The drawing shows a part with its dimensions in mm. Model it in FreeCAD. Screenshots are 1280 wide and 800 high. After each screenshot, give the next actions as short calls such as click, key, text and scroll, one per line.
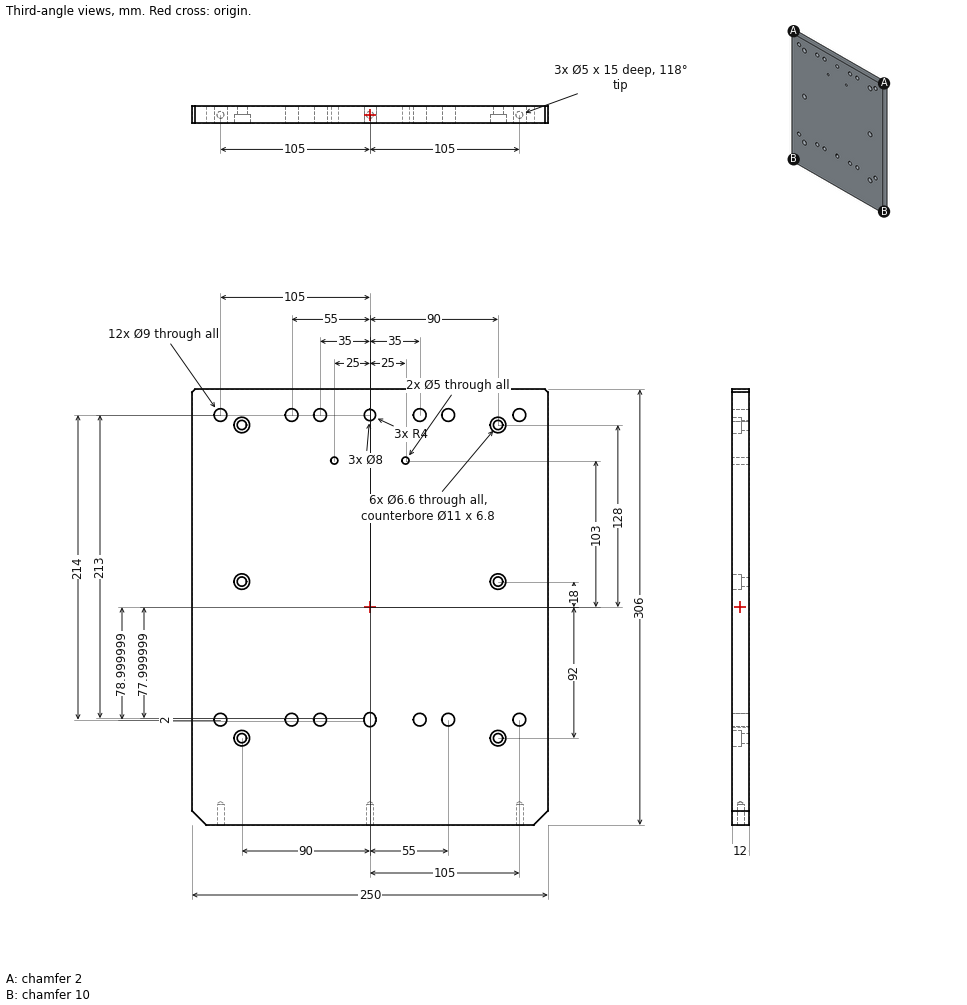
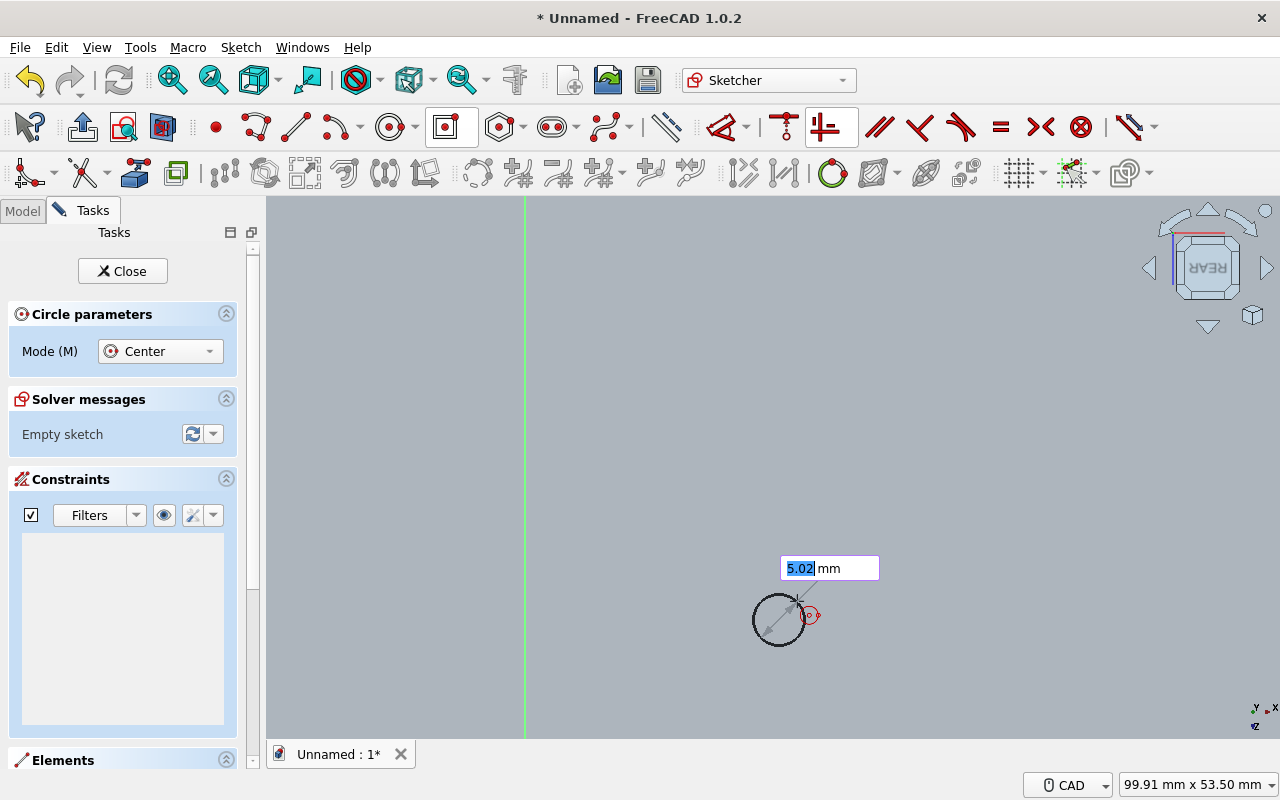
text(5)
key(Return)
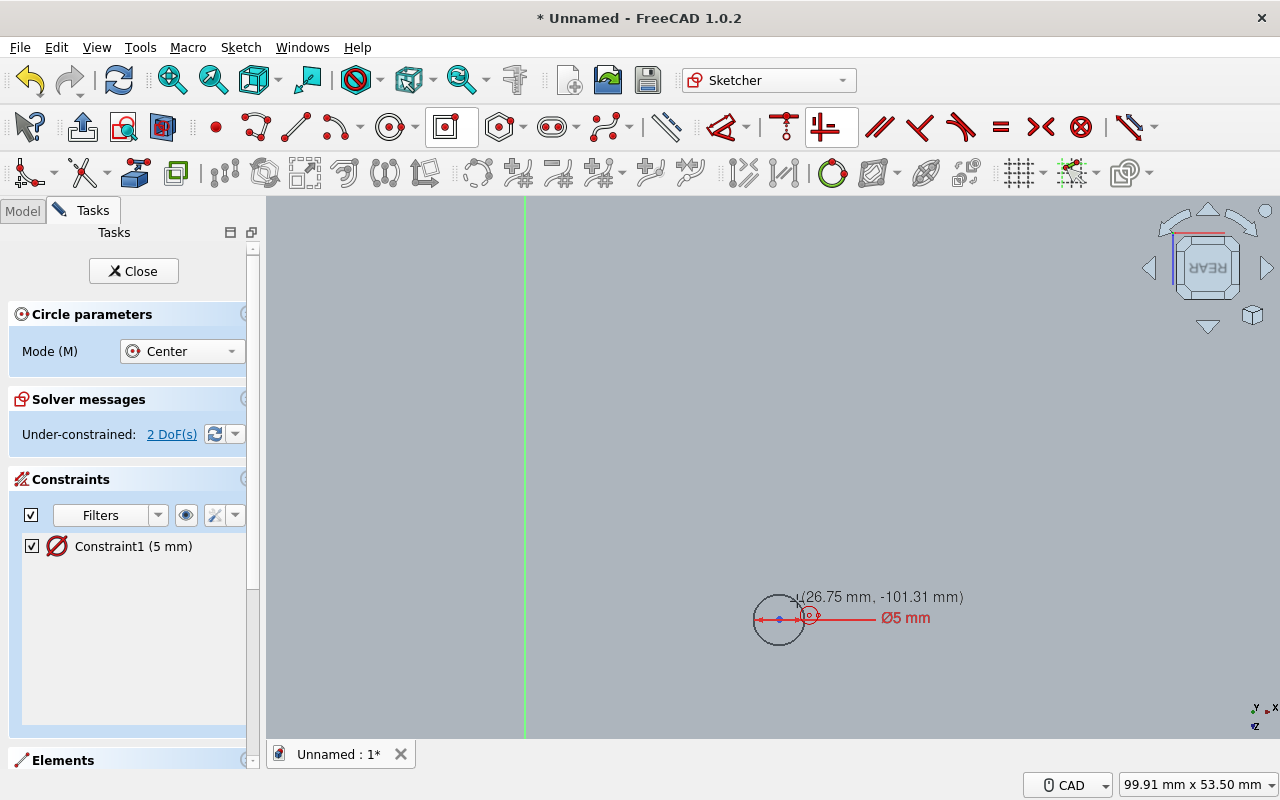
scroll(782, 622, down, 6)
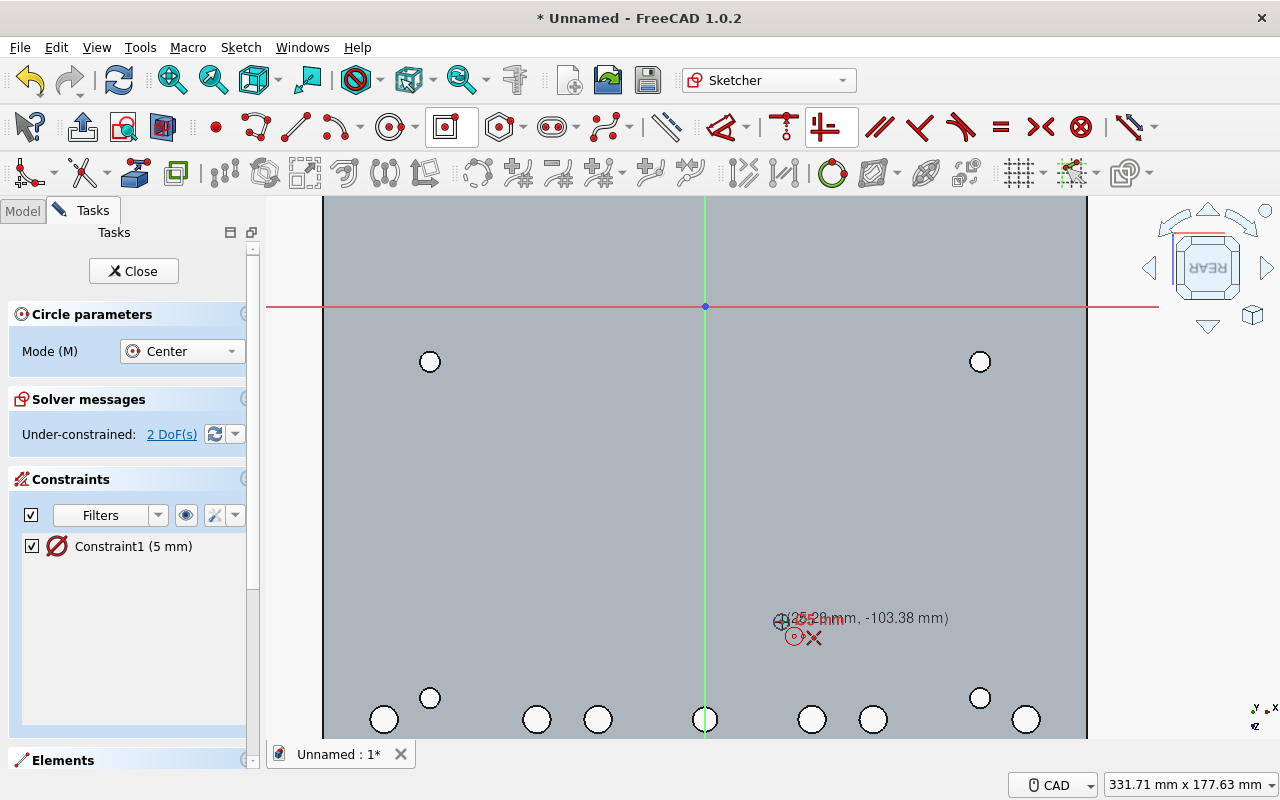
scroll(629, 622, up, 6)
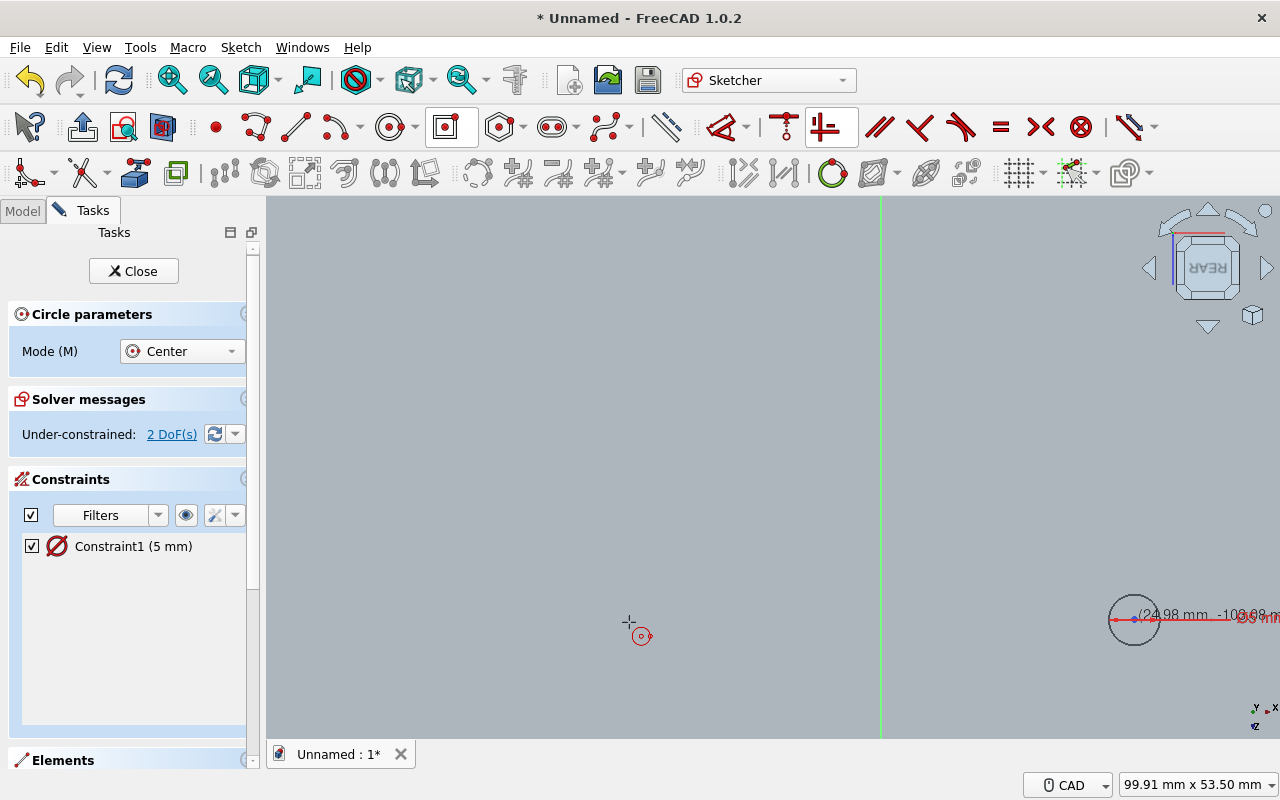
click(627, 619)
move(645, 601)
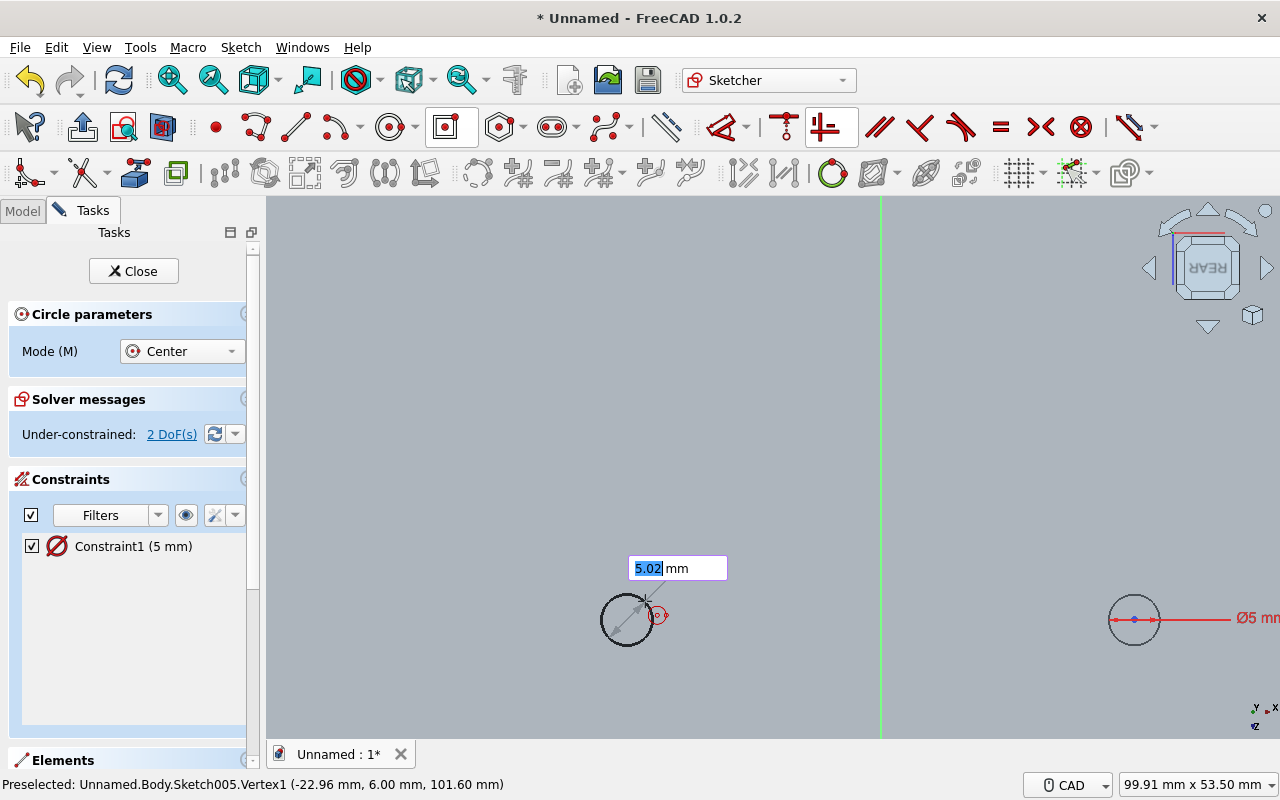
text(5)
key(Return)
key(Escape)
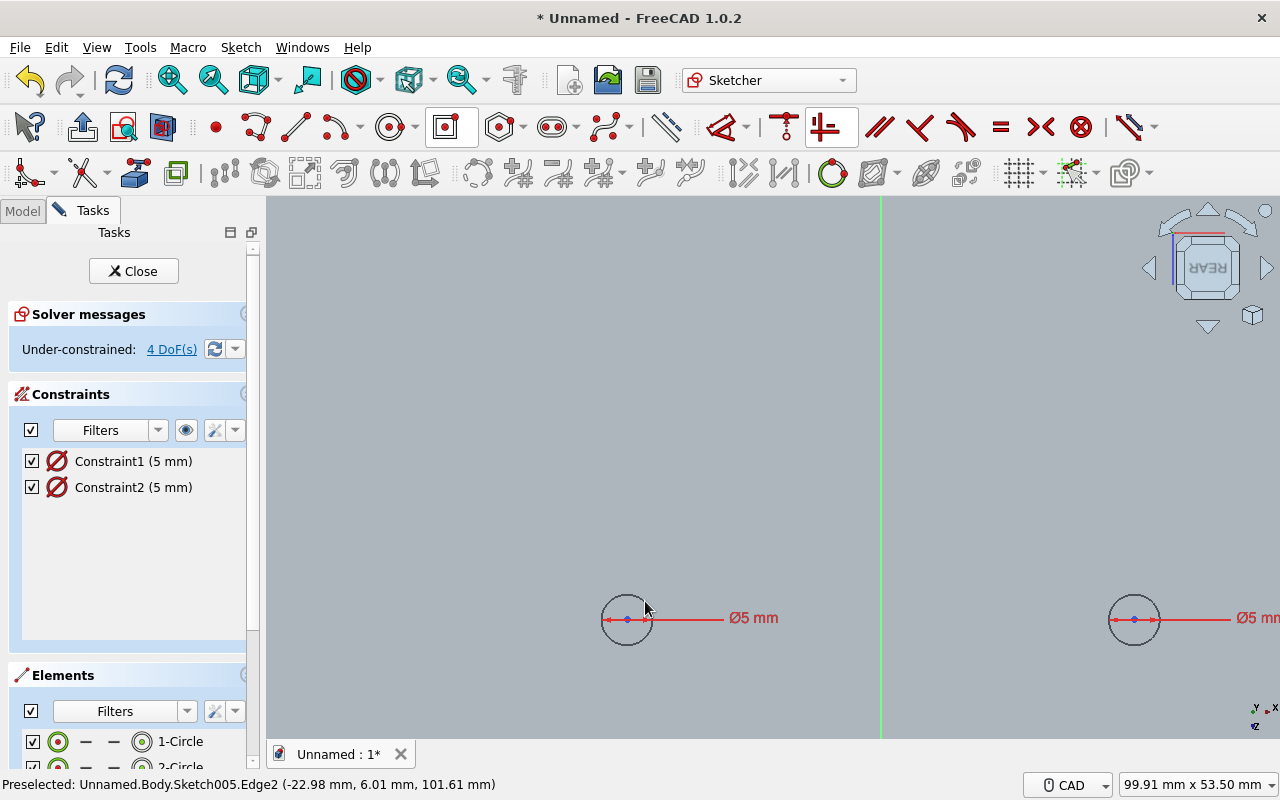
scroll(629, 622, down, 6)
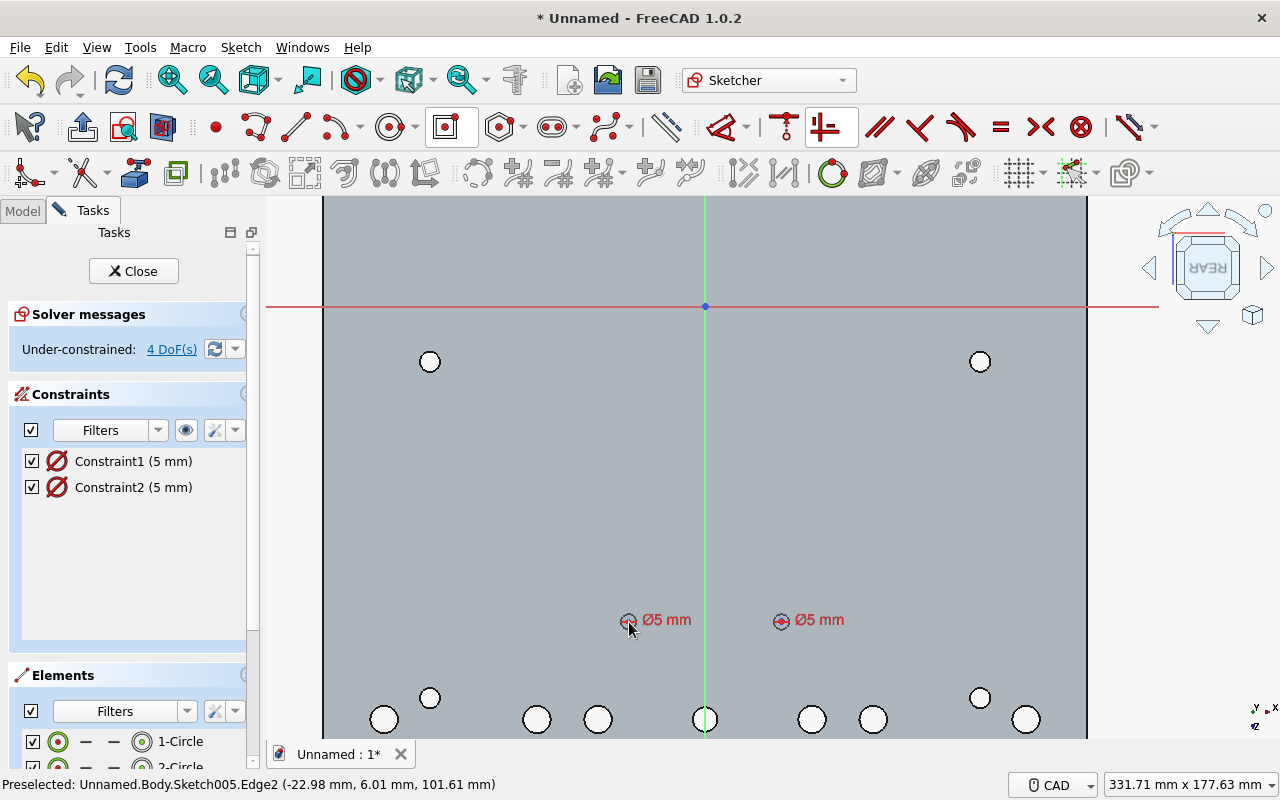
click(781, 622)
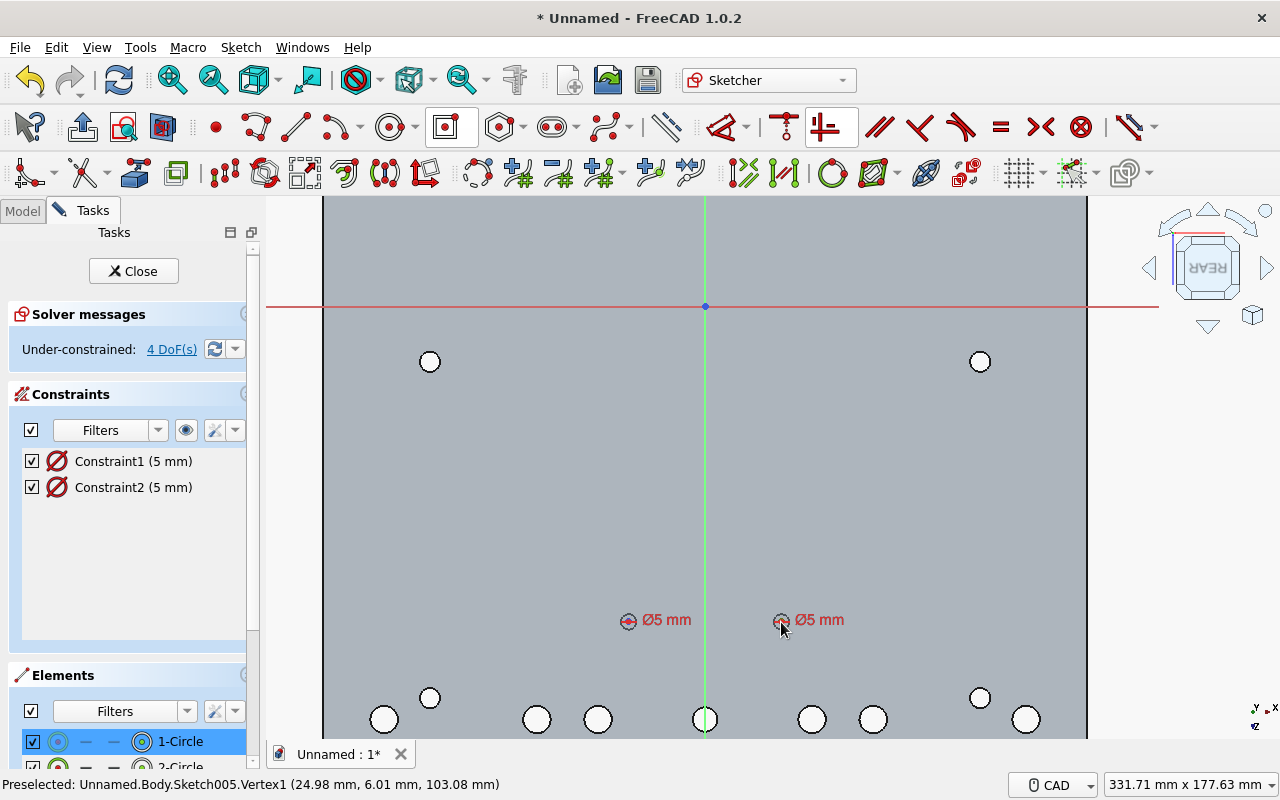
click(629, 622)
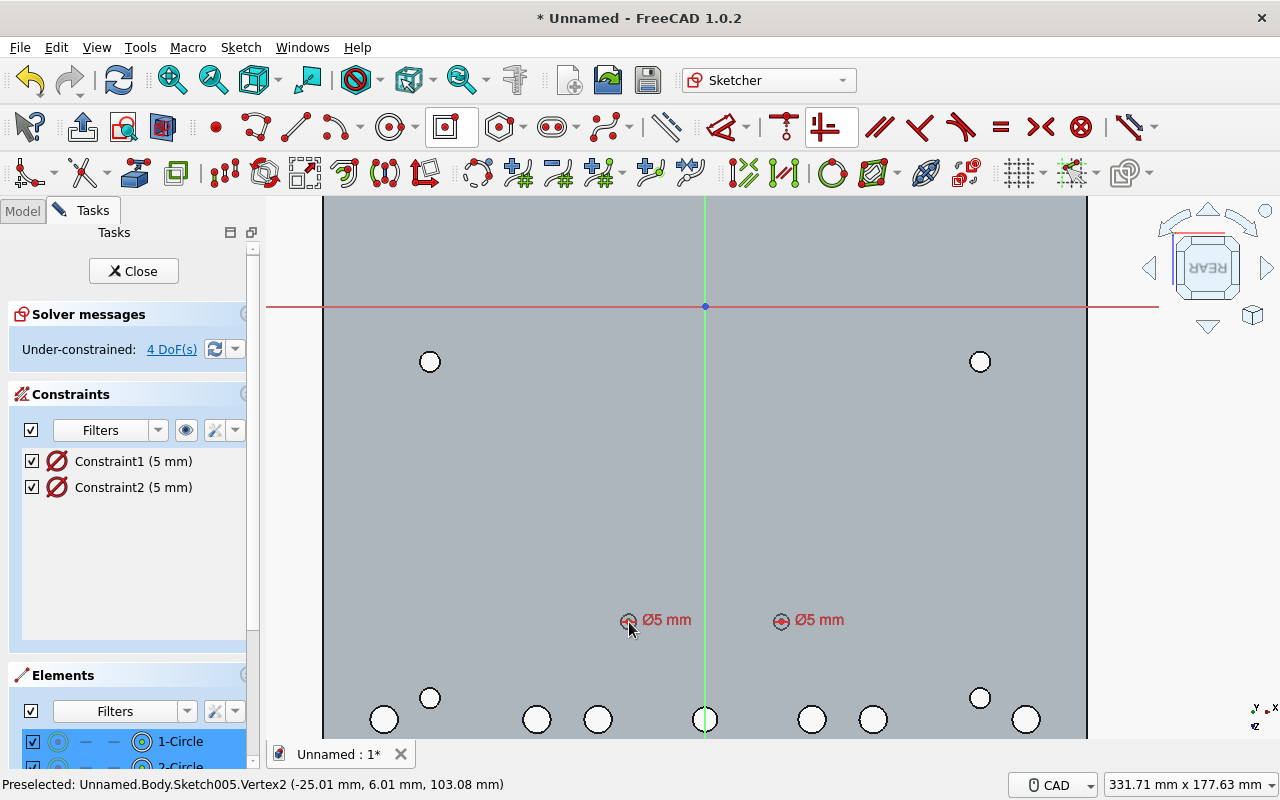
click(852, 128)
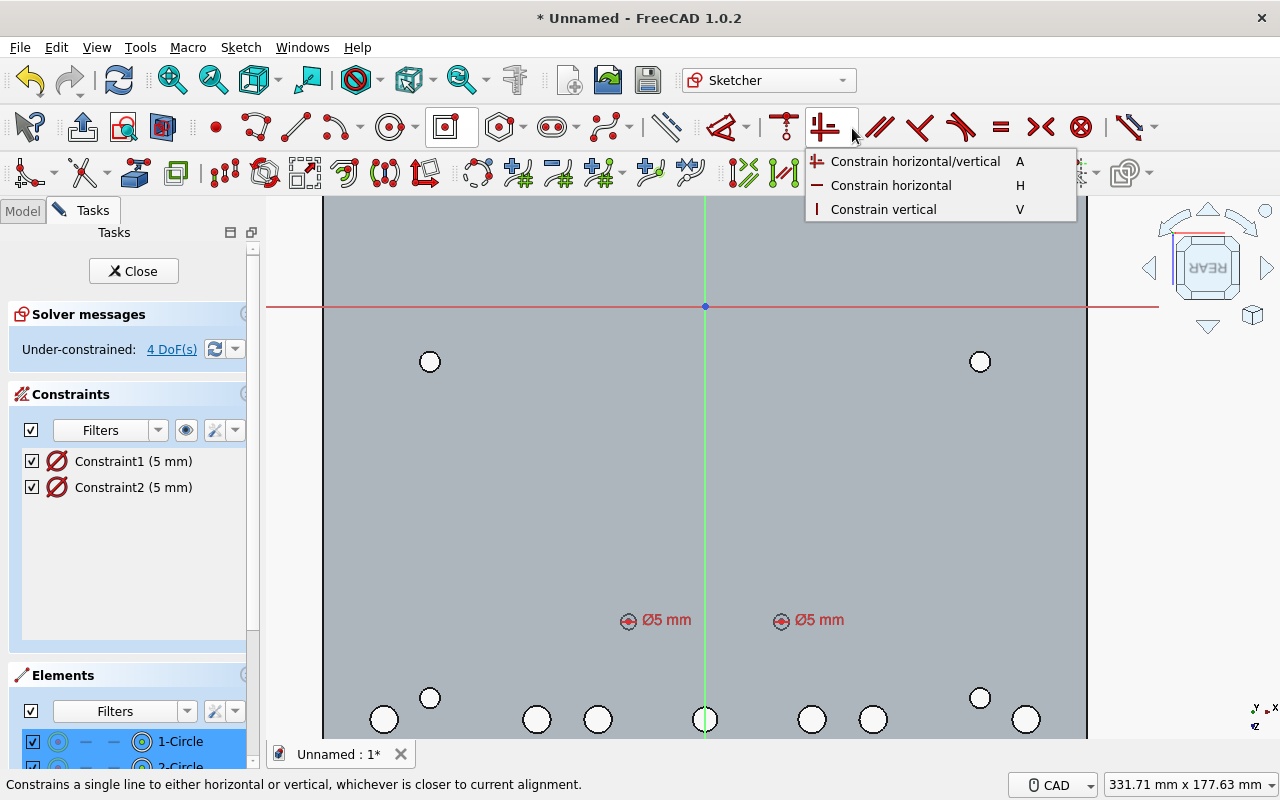
click(941, 185)